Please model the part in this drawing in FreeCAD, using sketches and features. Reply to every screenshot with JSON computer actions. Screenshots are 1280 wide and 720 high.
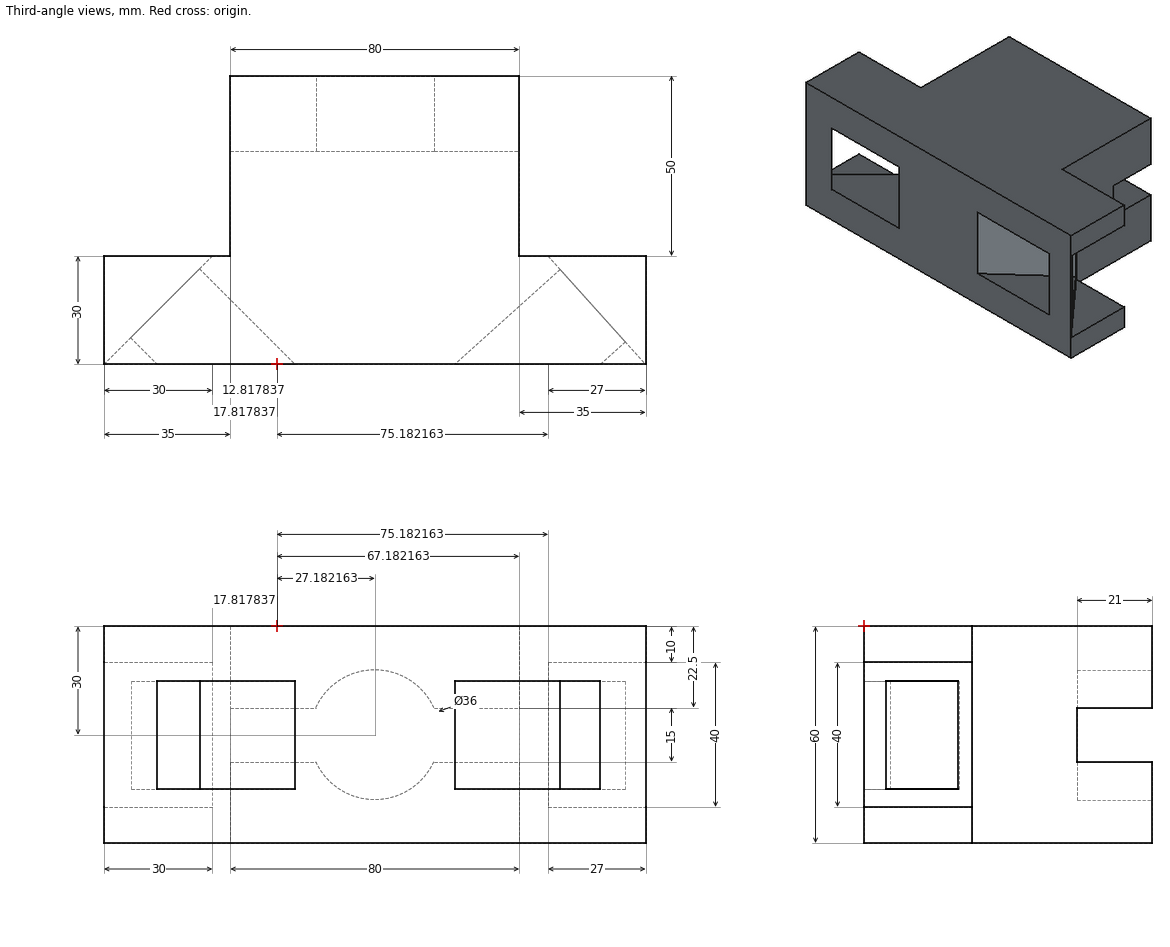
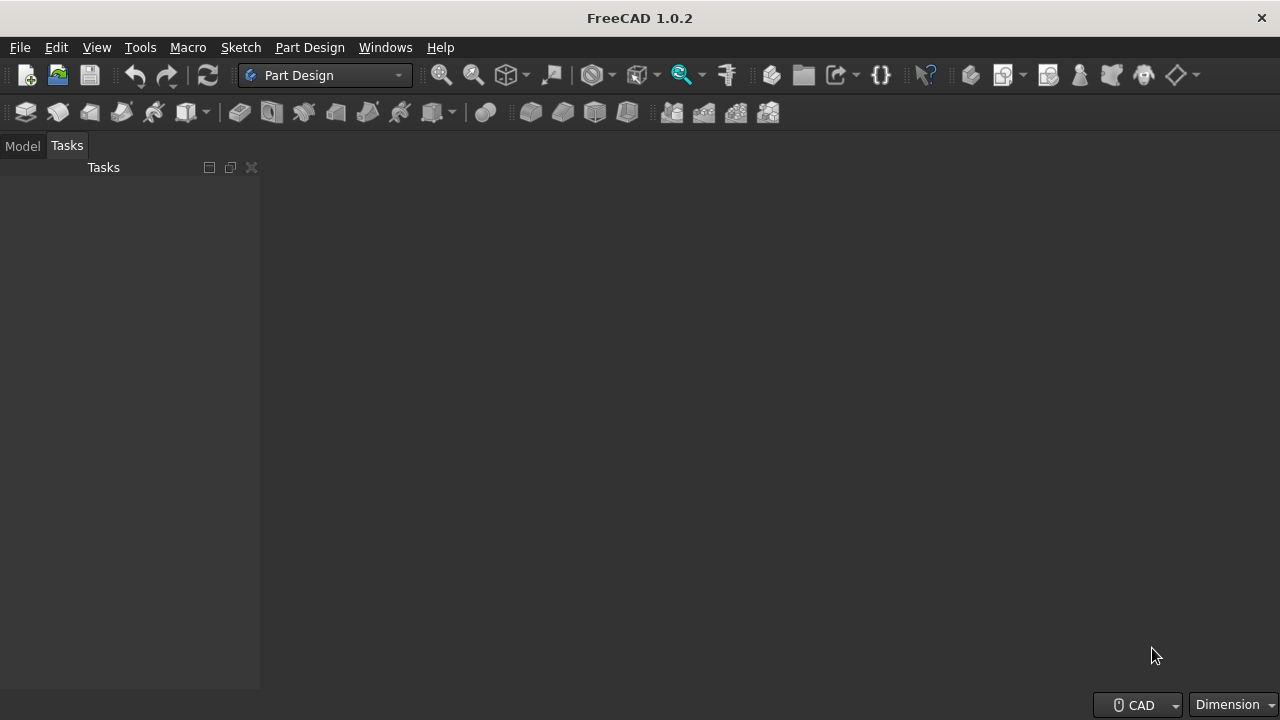
{"action": "left_click", "coordinate": [26, 76]}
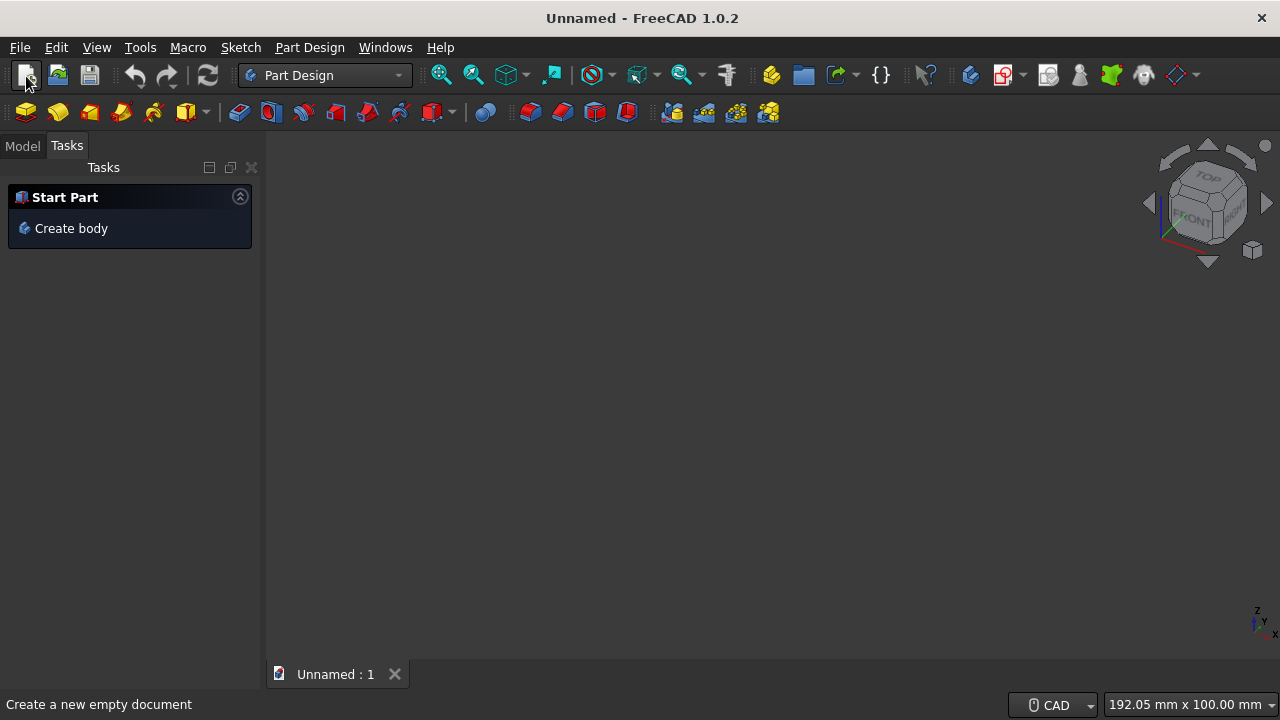
{"action": "left_click", "coordinate": [1004, 76]}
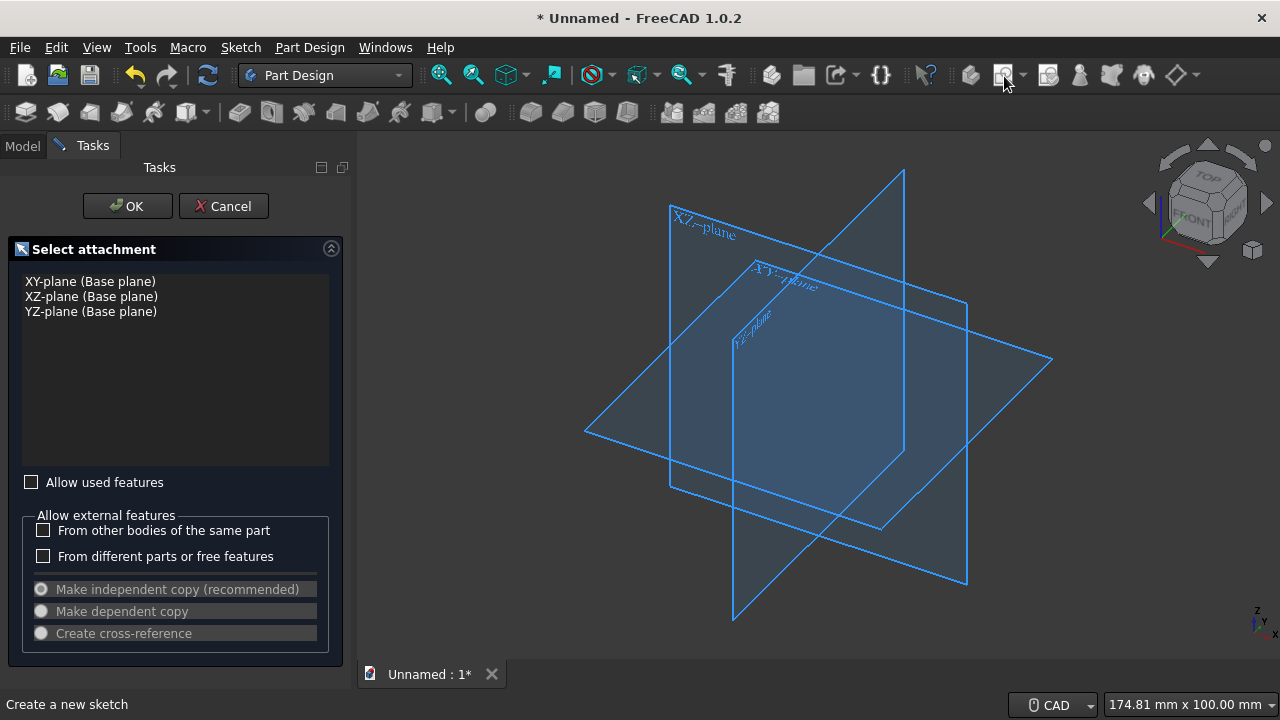
{"action": "left_click", "coordinate": [82, 282]}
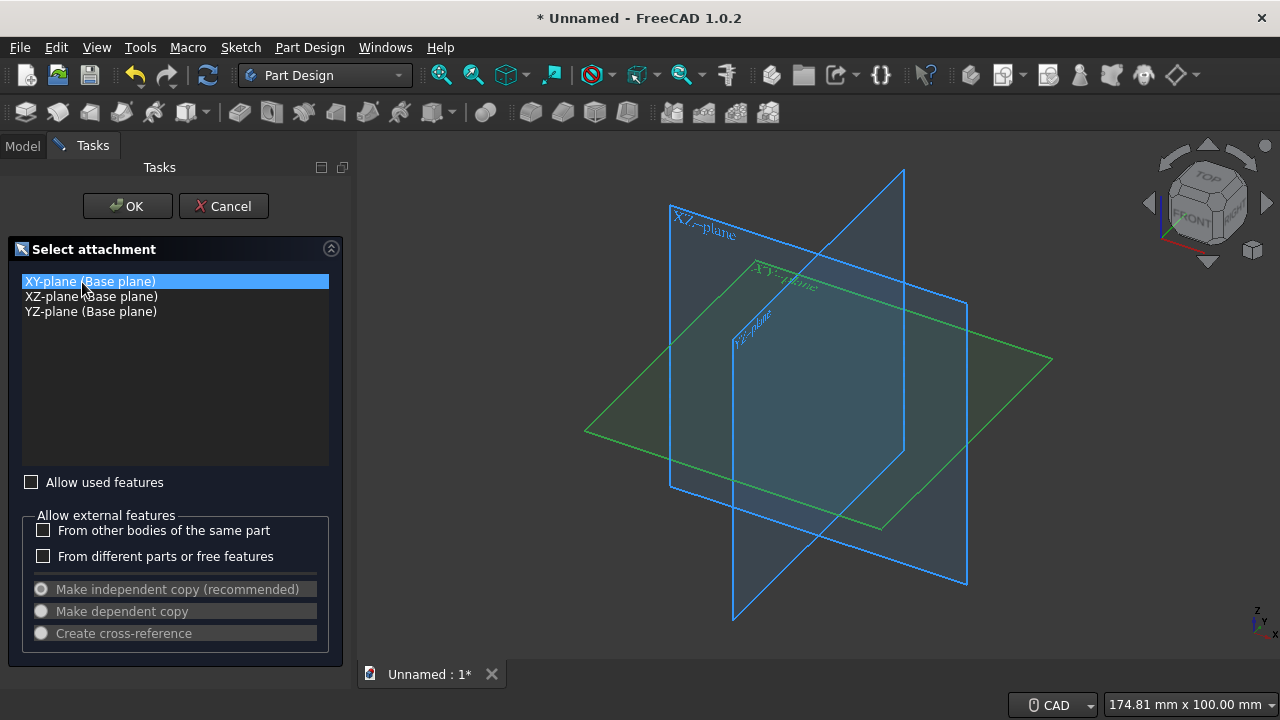
{"action": "left_click", "coordinate": [128, 206]}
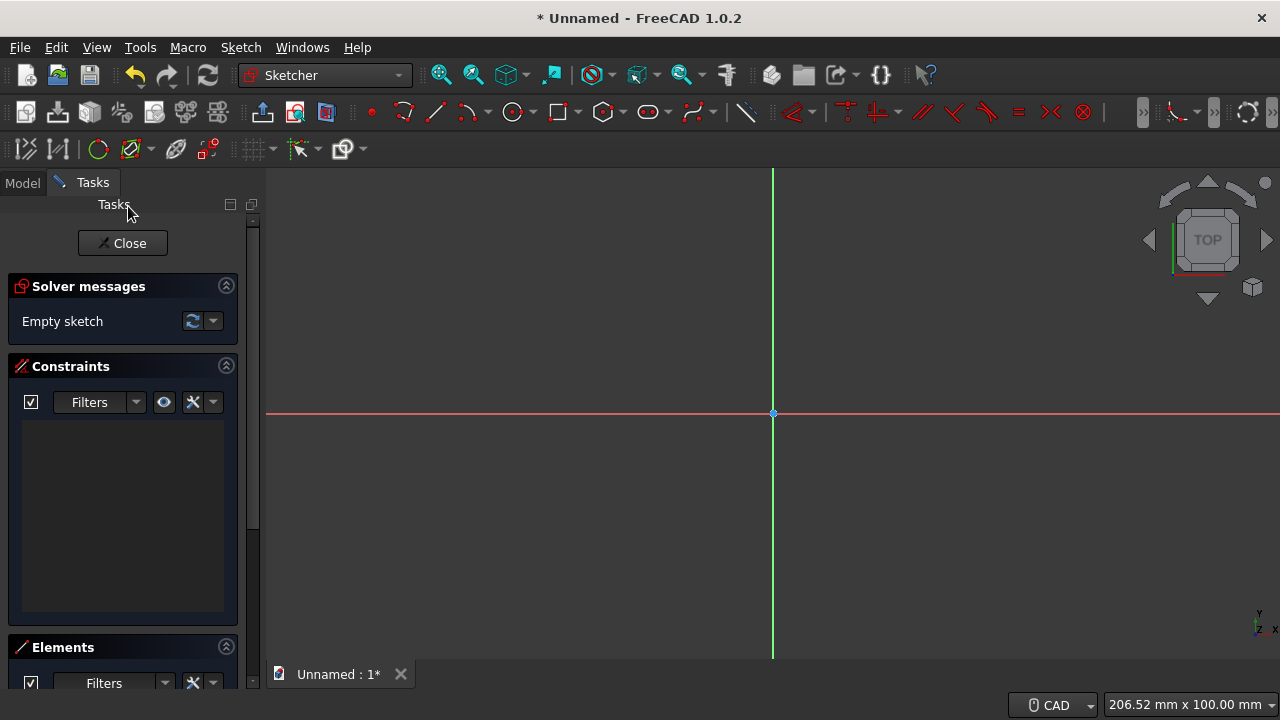
{"action": "scroll", "coordinate": [294, 631], "scroll_direction": "down", "scroll_amount": 2}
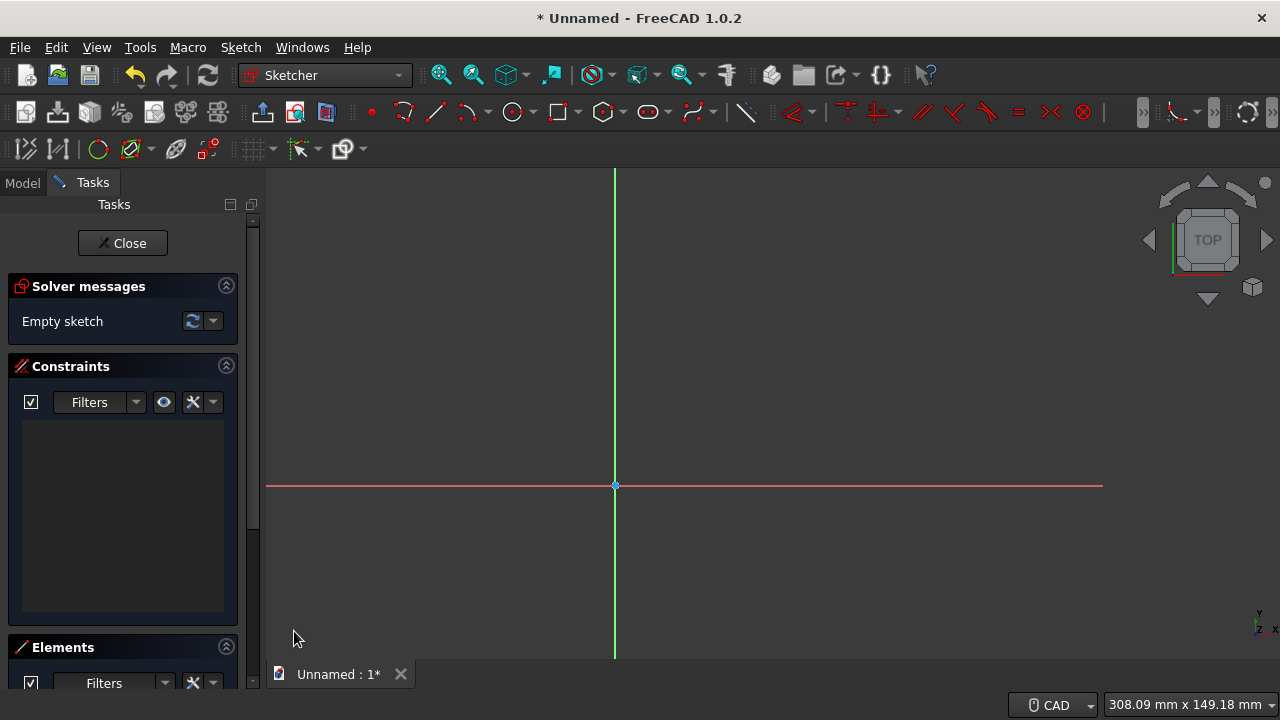
{"action": "left_click", "coordinate": [404, 112]}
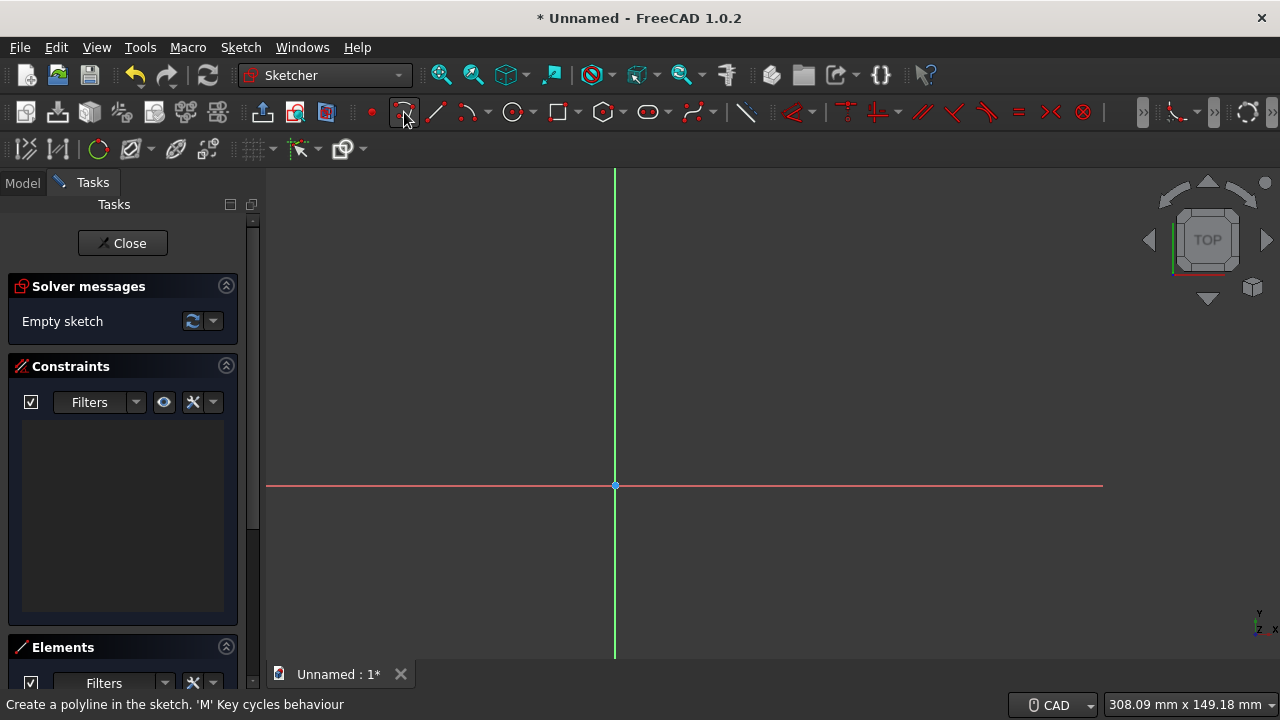
{"action": "left_click", "coordinate": [573, 387]}
{"action": "left_click", "coordinate": [458, 387]}
{"action": "left_click", "coordinate": [458, 486]}
{"action": "left_click", "coordinate": [951, 477]}
{"action": "left_click", "coordinate": [951, 387]}
{"action": "left_click", "coordinate": [836, 387]}
{"action": "left_click", "coordinate": [836, 222]}
{"action": "left_click", "coordinate": [573, 222]}
{"action": "left_click", "coordinate": [573, 388]}
{"action": "key", "text": "Escape"}
{"action": "key", "text": "Escape"}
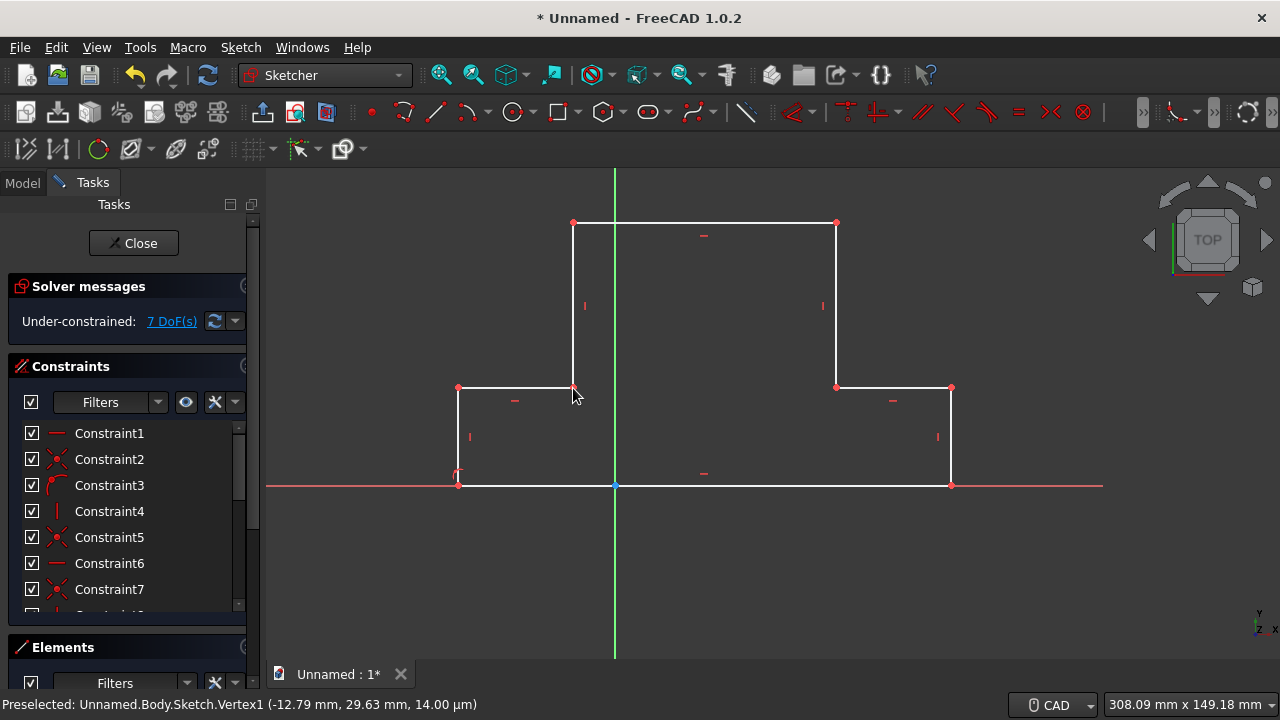
{"action": "left_click", "coordinate": [792, 112]}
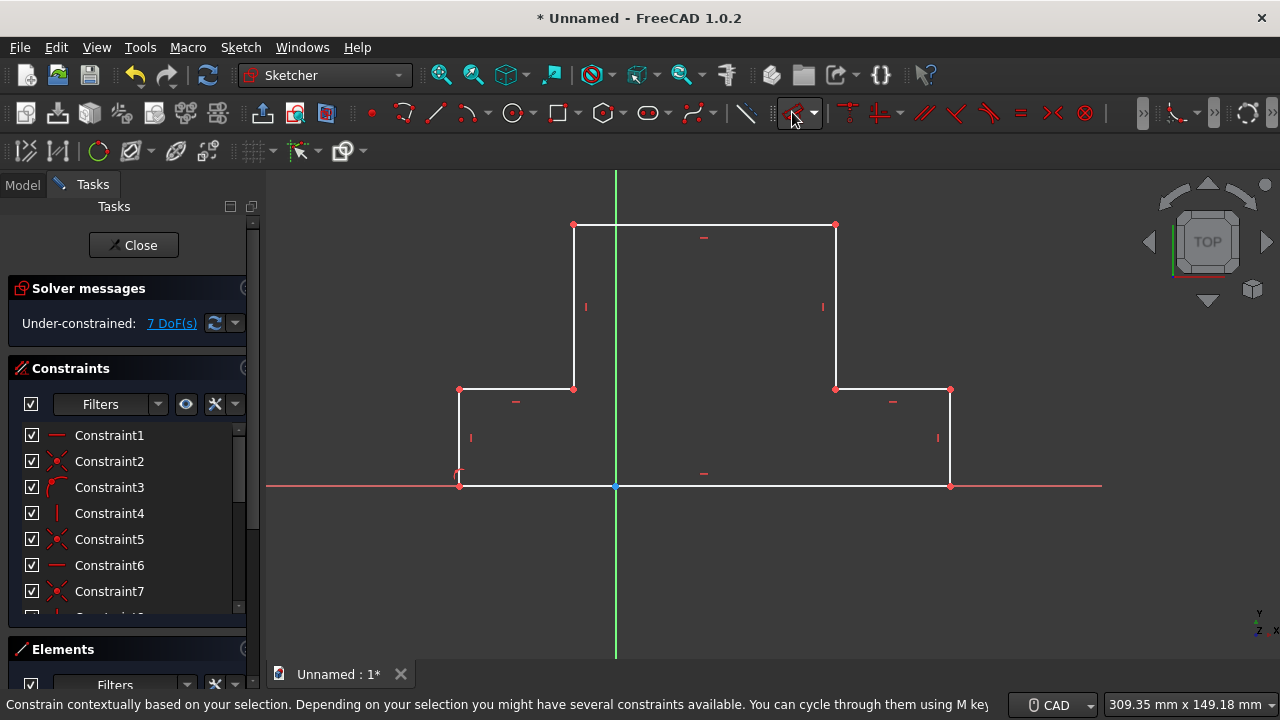
{"action": "left_click", "coordinate": [539, 389]}
{"action": "left_click", "coordinate": [517, 423]}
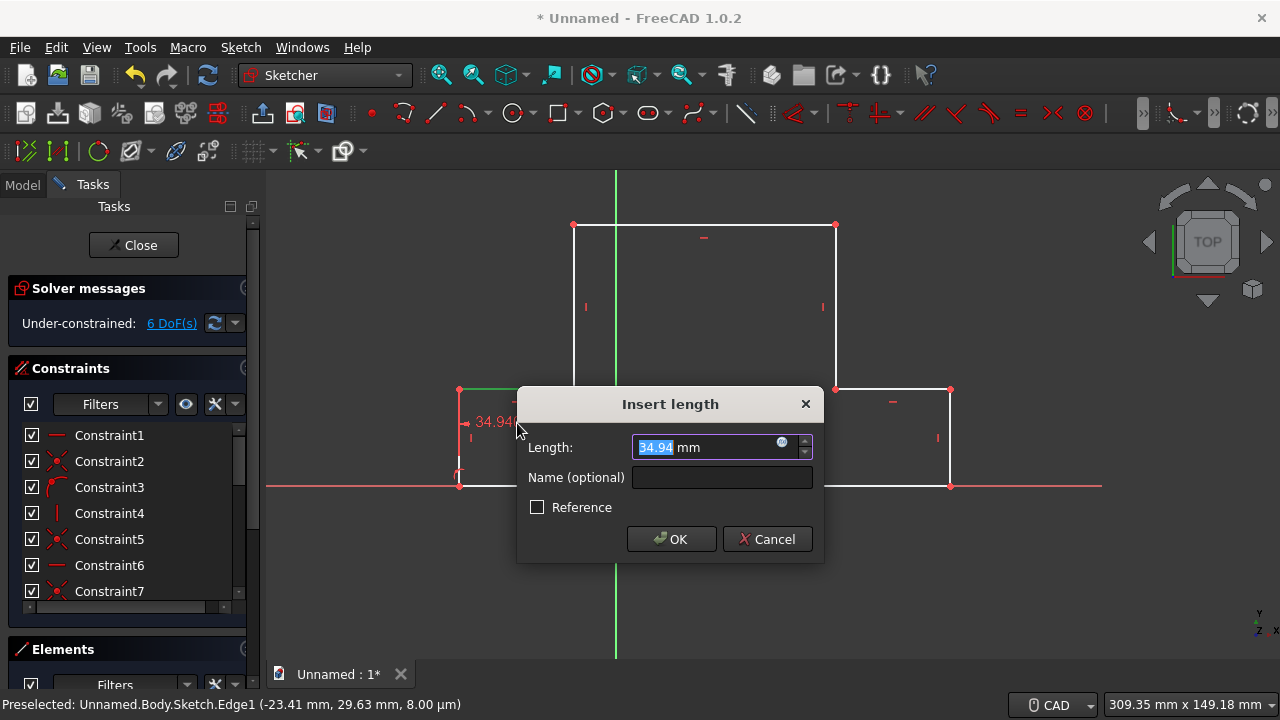
{"action": "type", "text": "35"}
{"action": "key", "text": "Return"}